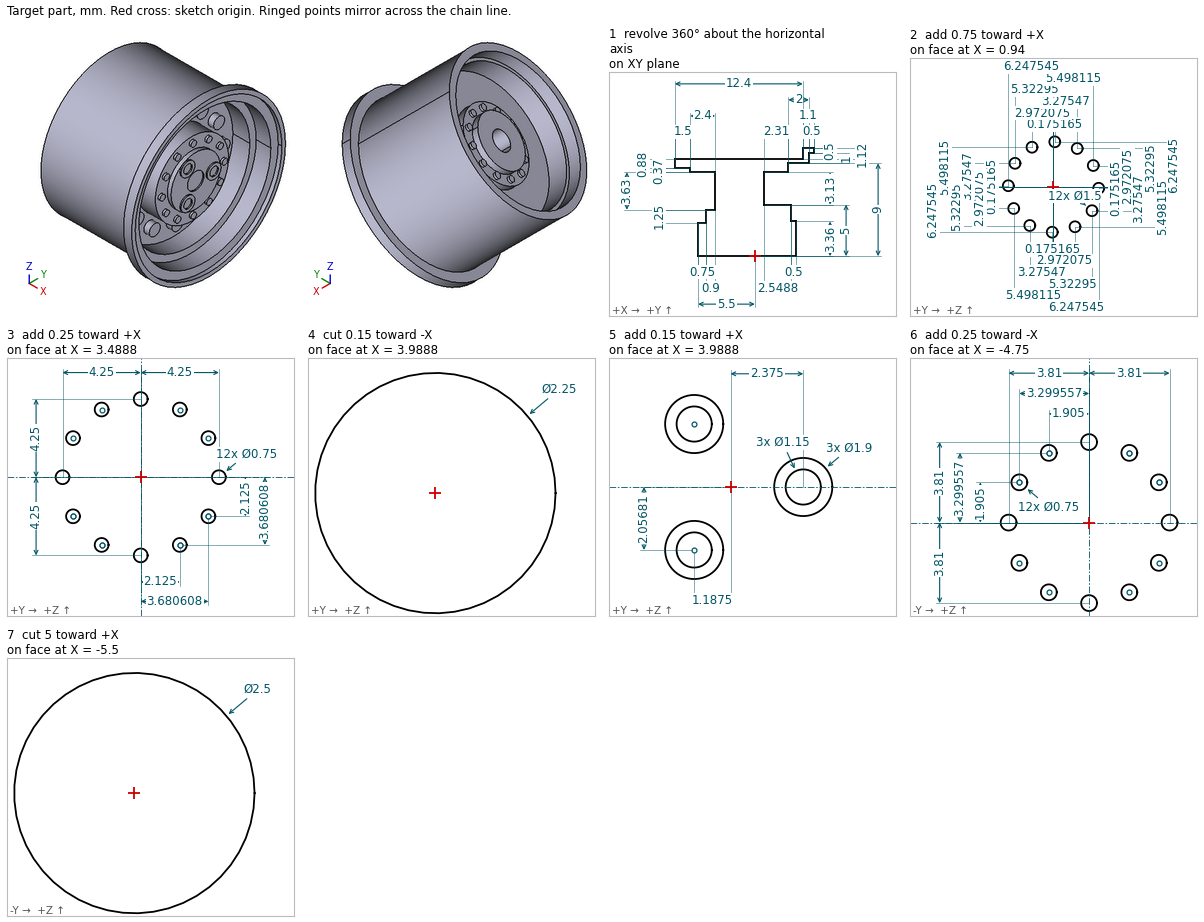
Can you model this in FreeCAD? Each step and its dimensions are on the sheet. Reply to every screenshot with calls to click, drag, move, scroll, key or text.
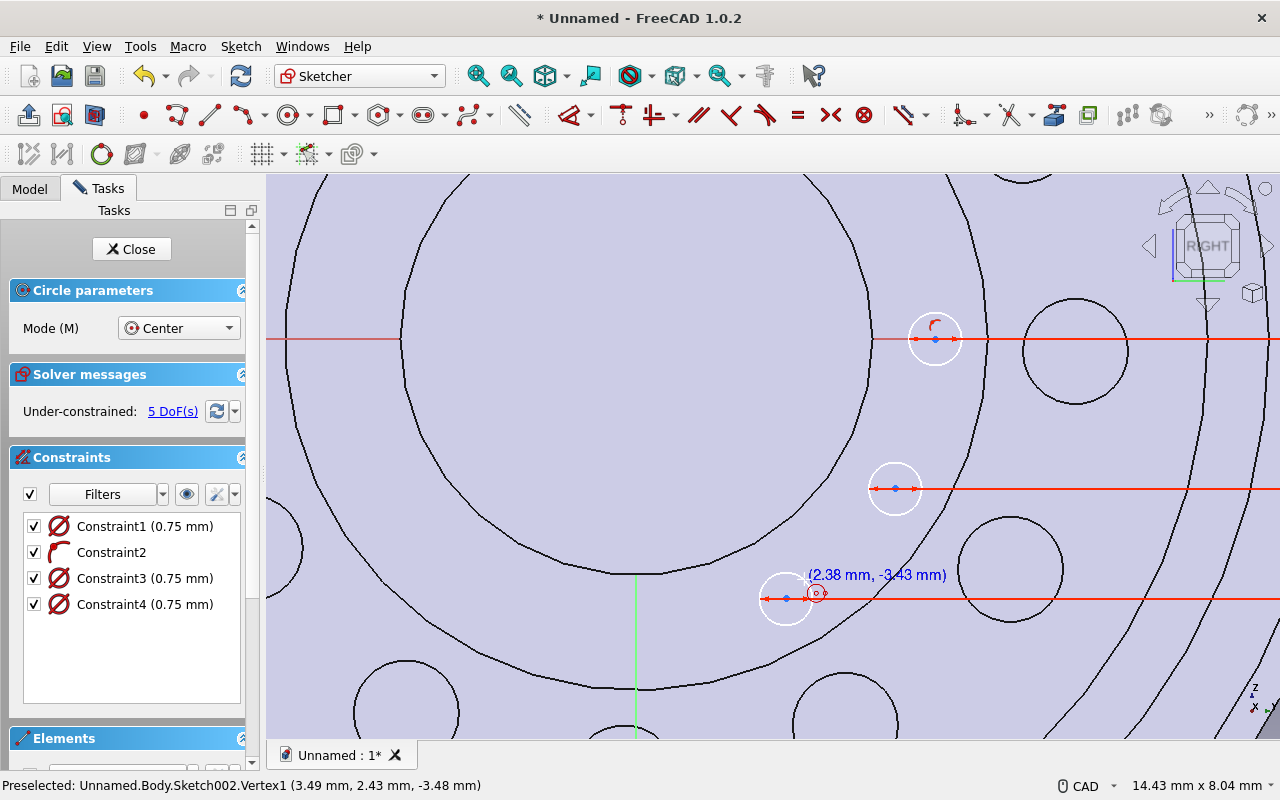
click(636, 638)
move(655, 619)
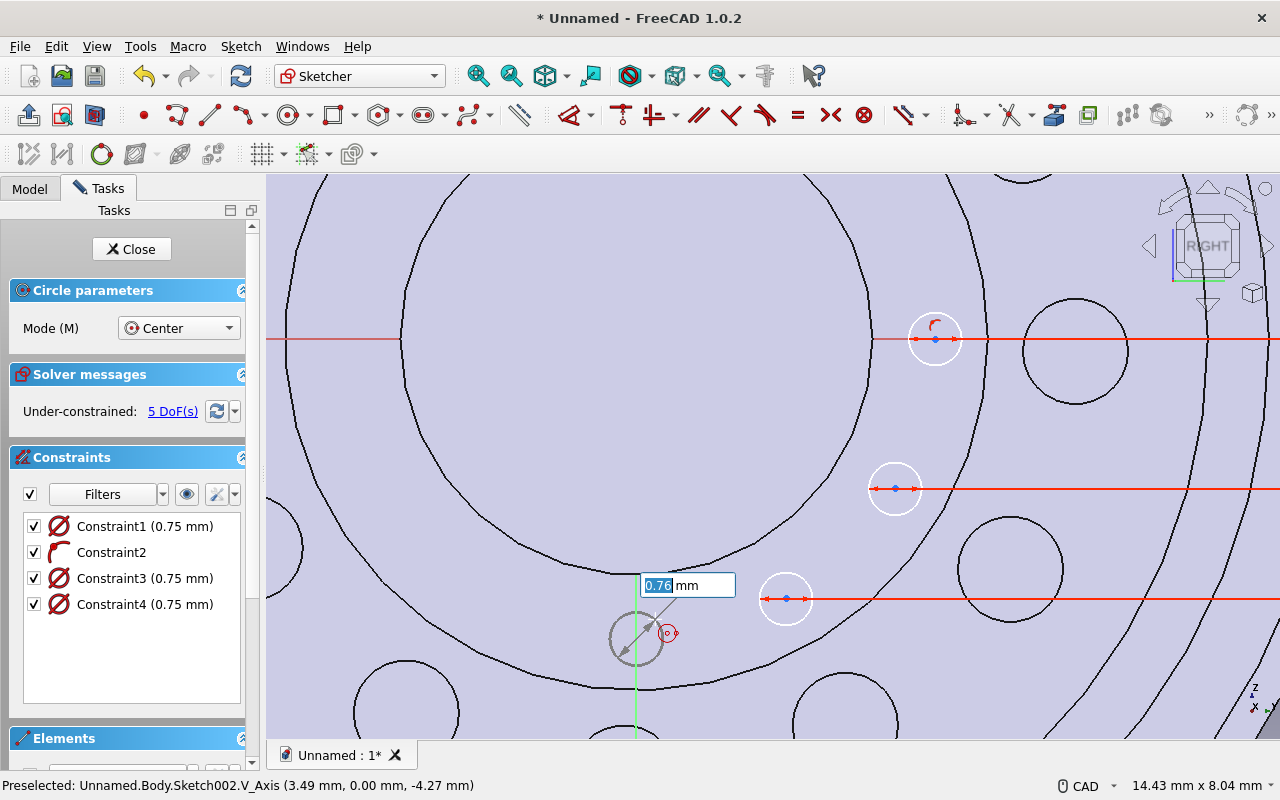
text(0.75)
key(Return)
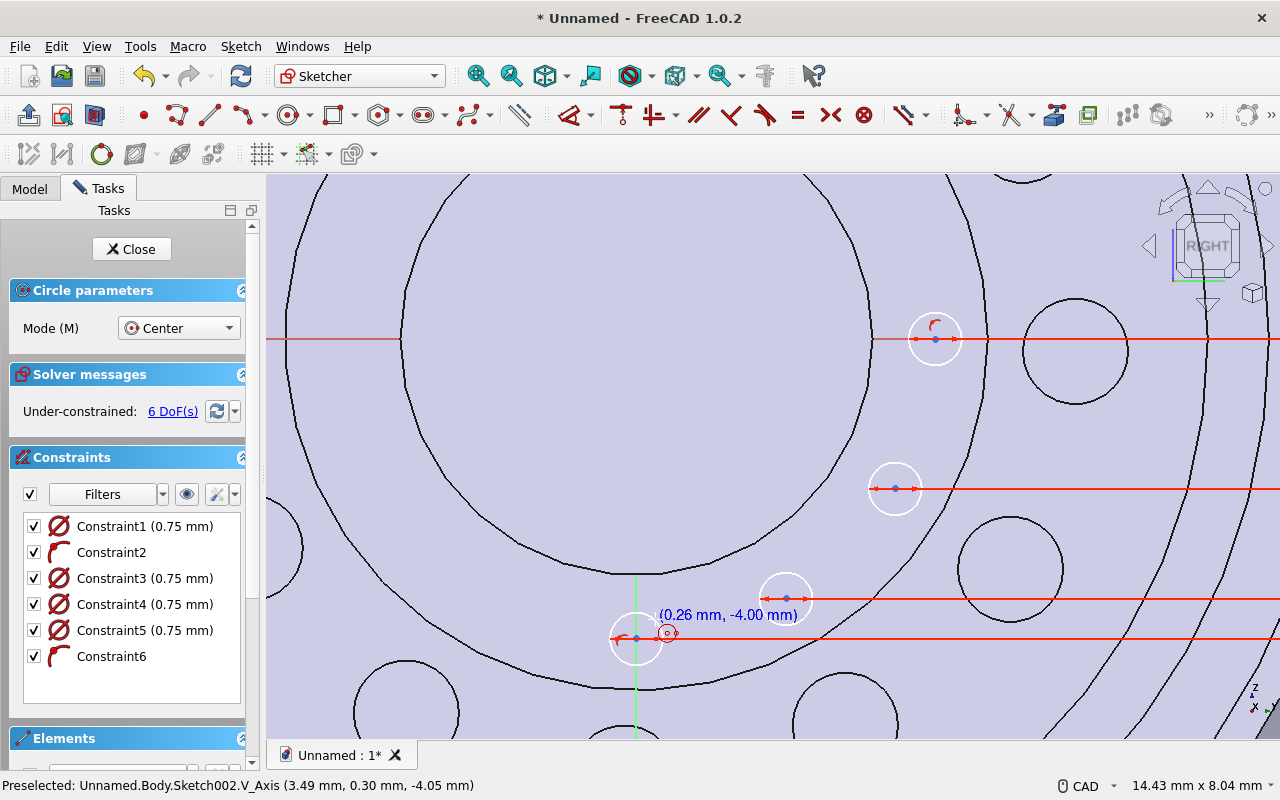
click(487, 598)
move(506, 579)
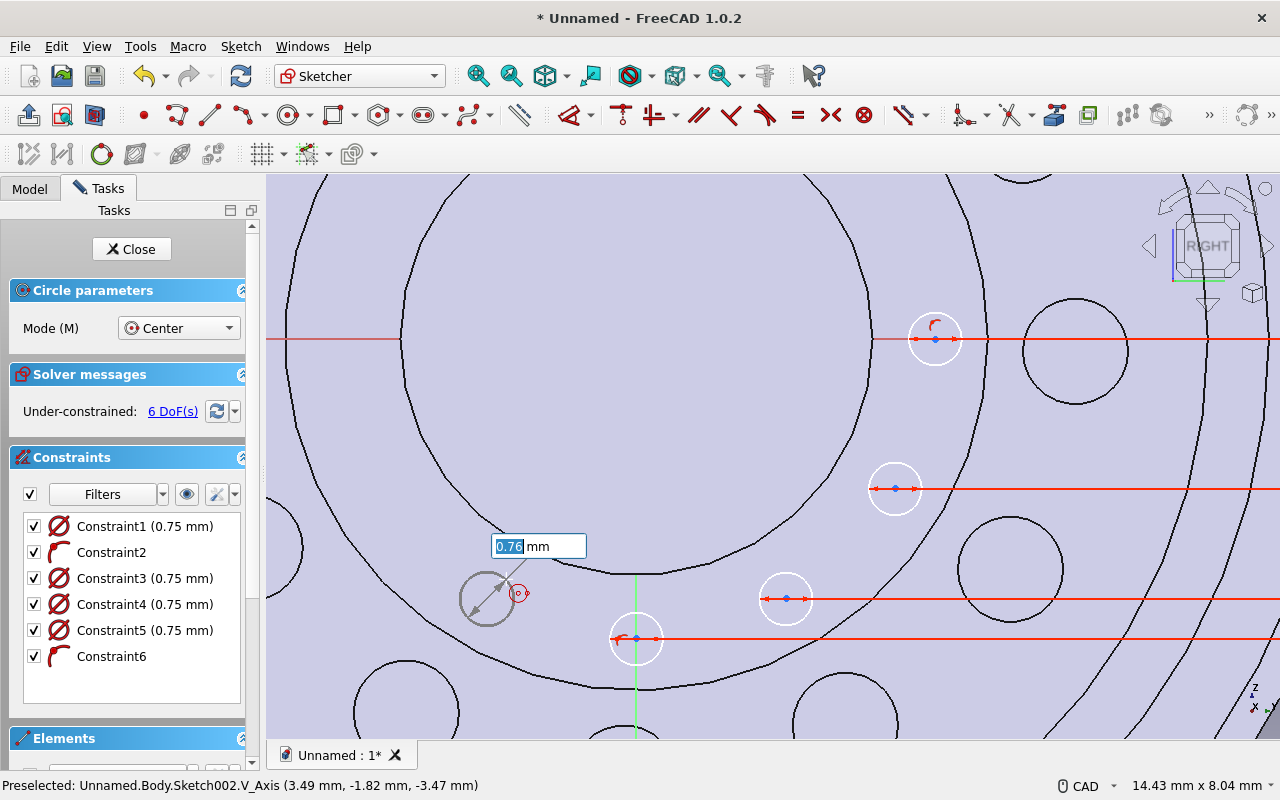
text(0.75)
key(Return)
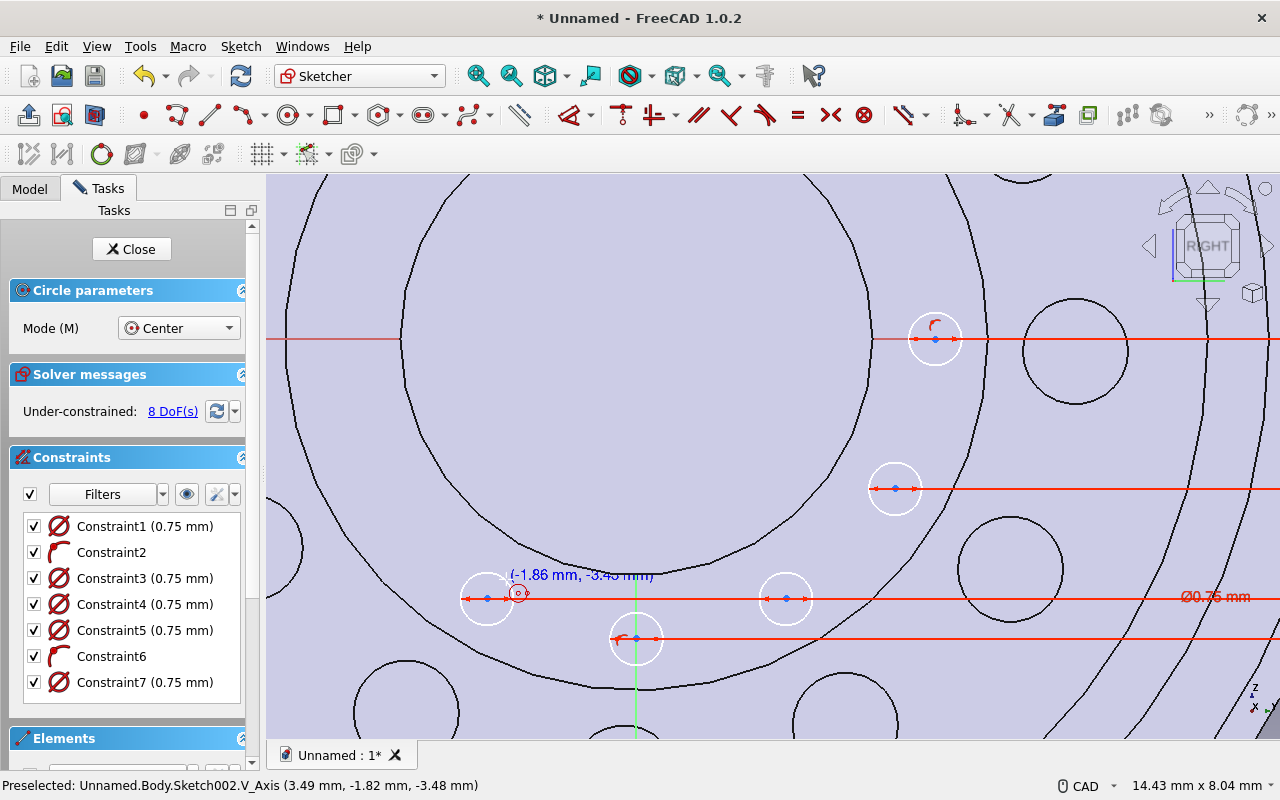
click(378, 488)
move(396, 470)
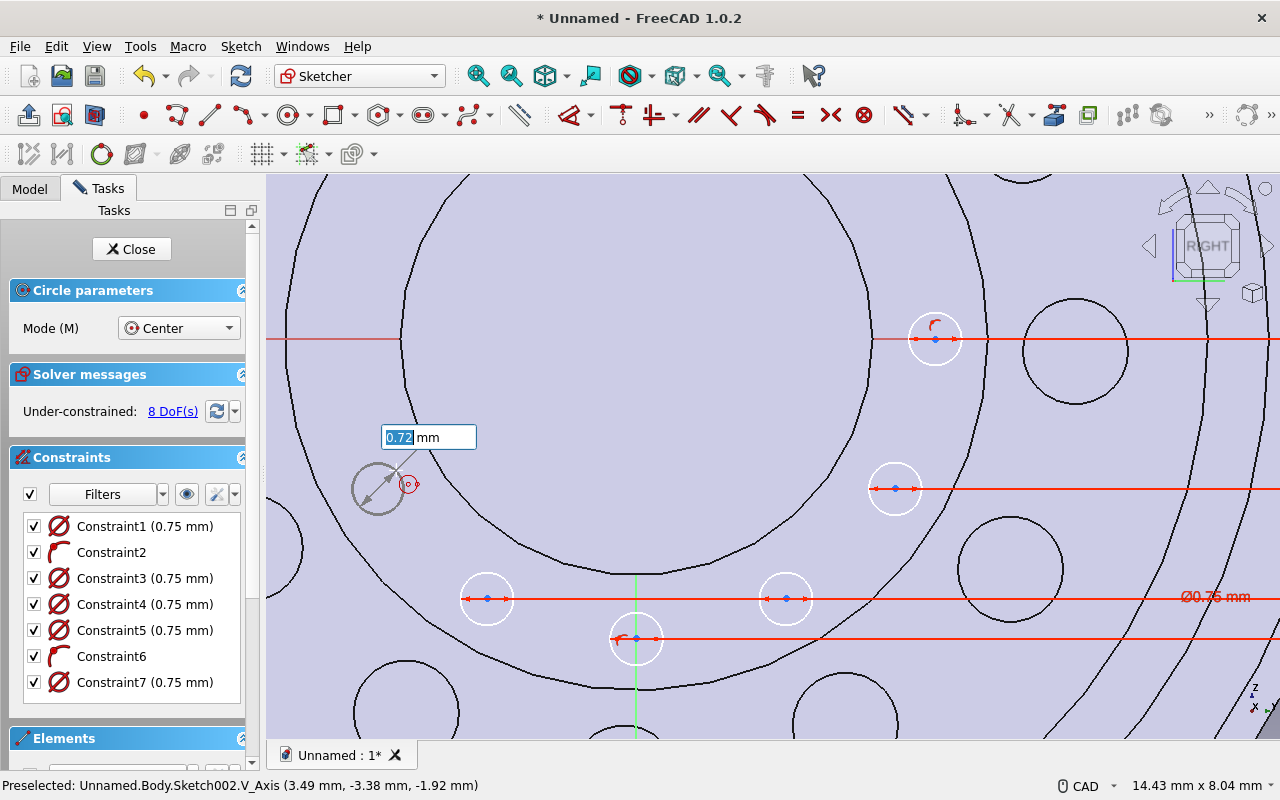
text(0.75)
key(Return)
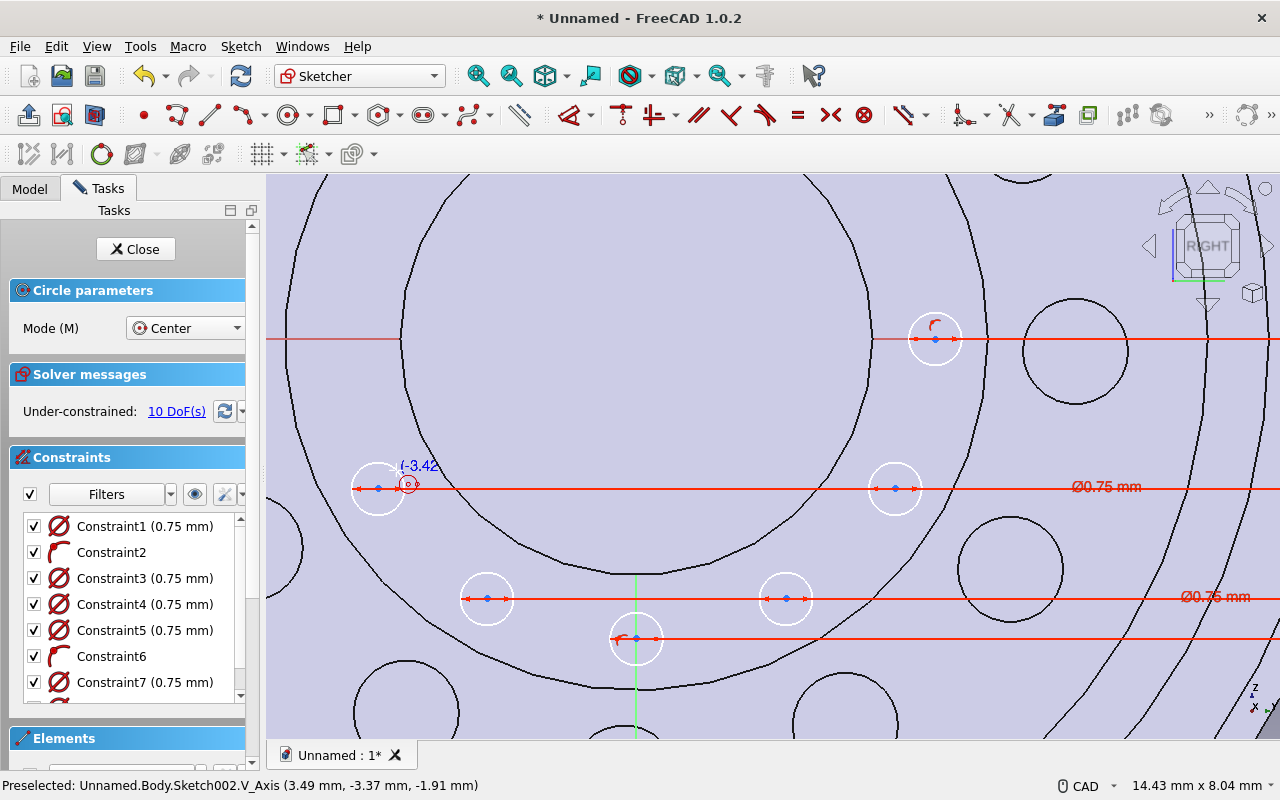
click(338, 339)
move(356, 320)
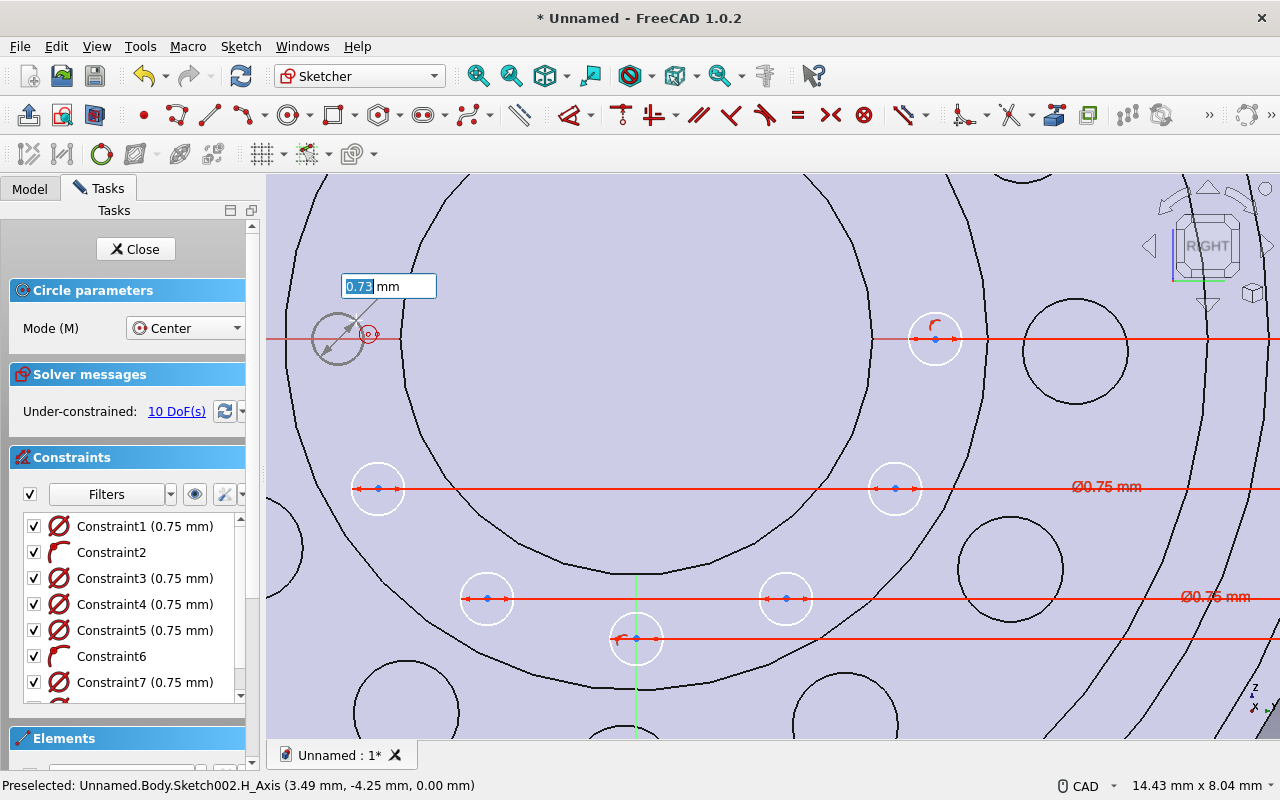
text(0.75)
key(Return)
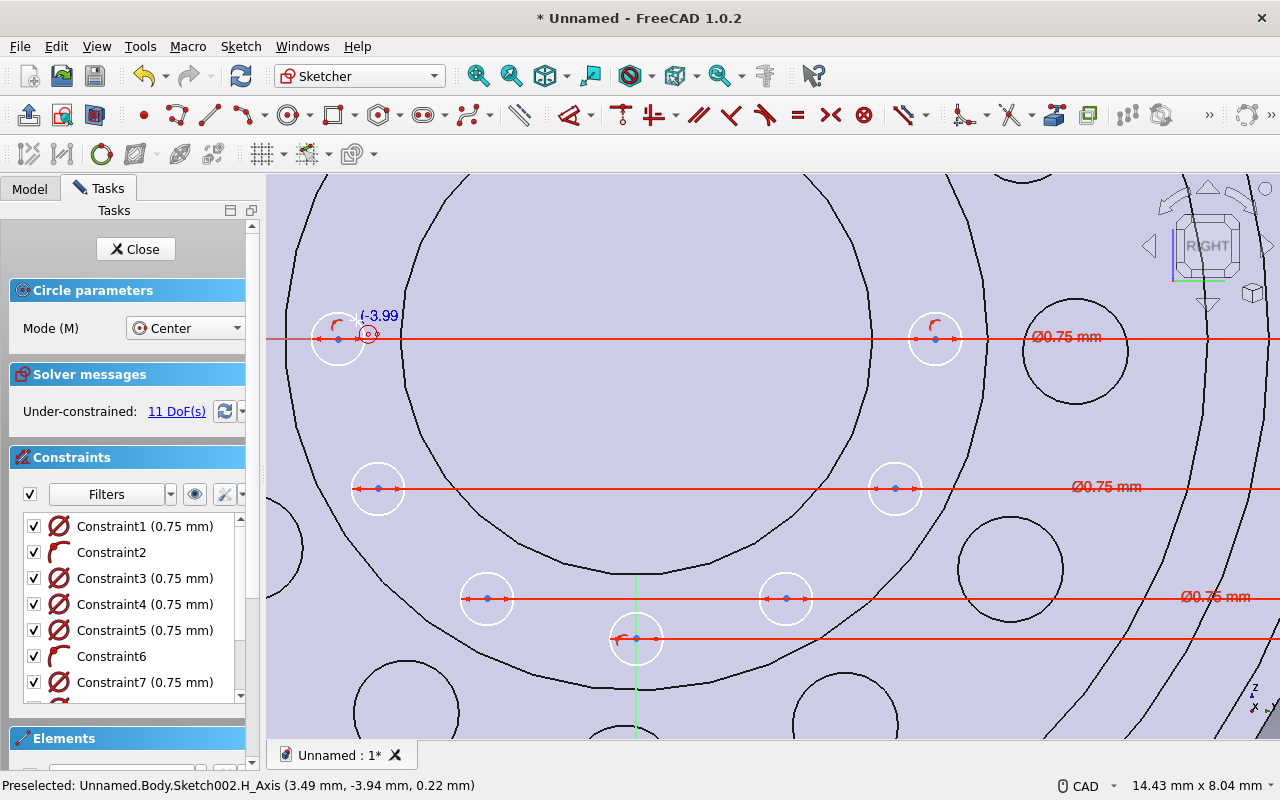
scroll(787, 599, down, 3)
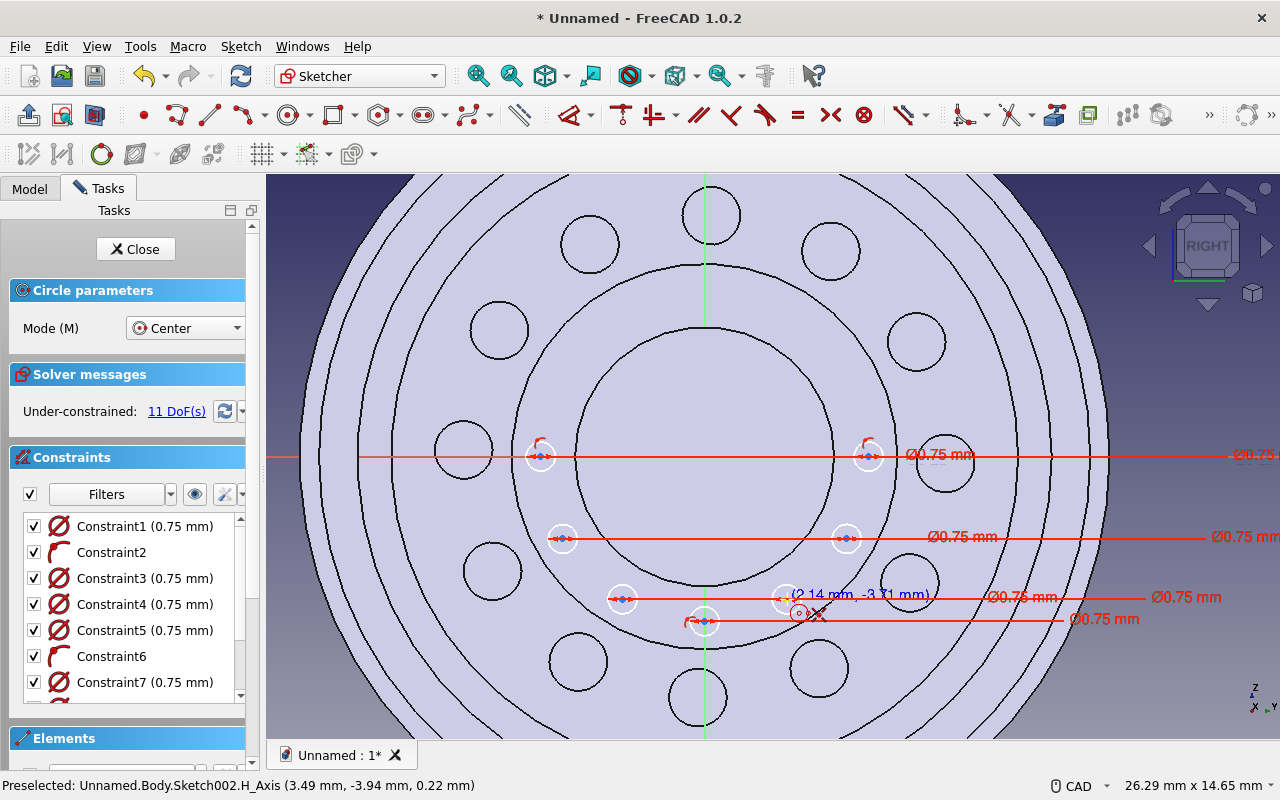
scroll(563, 375, up, 3)